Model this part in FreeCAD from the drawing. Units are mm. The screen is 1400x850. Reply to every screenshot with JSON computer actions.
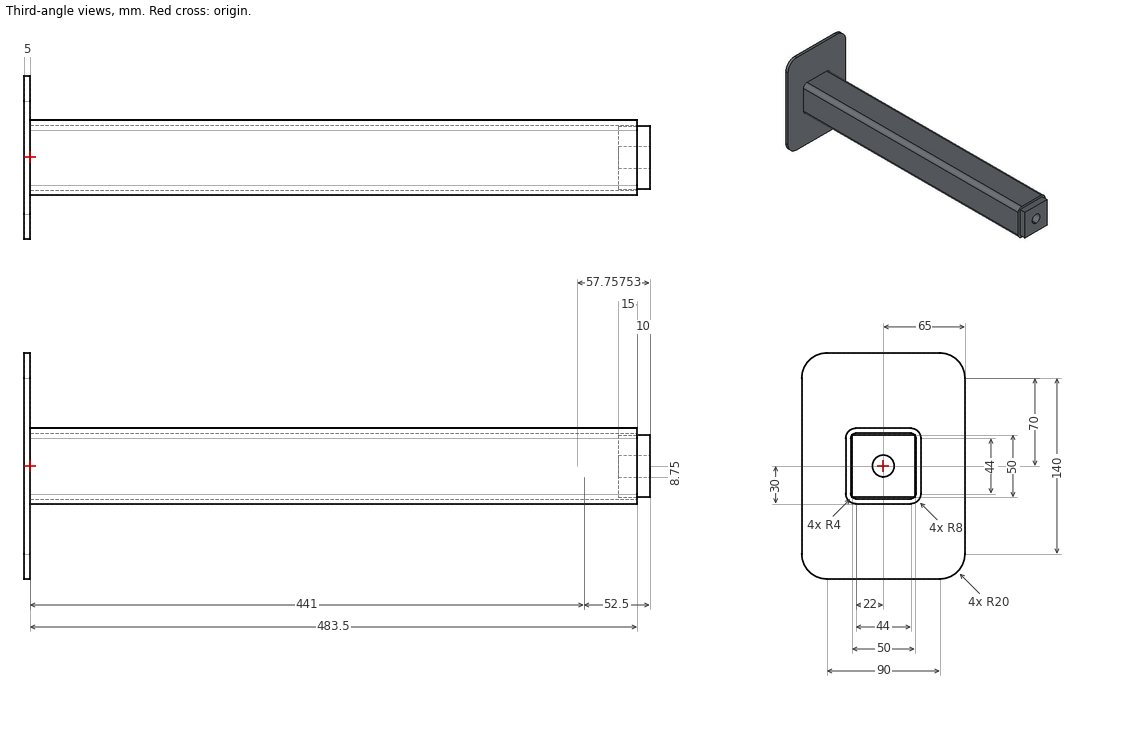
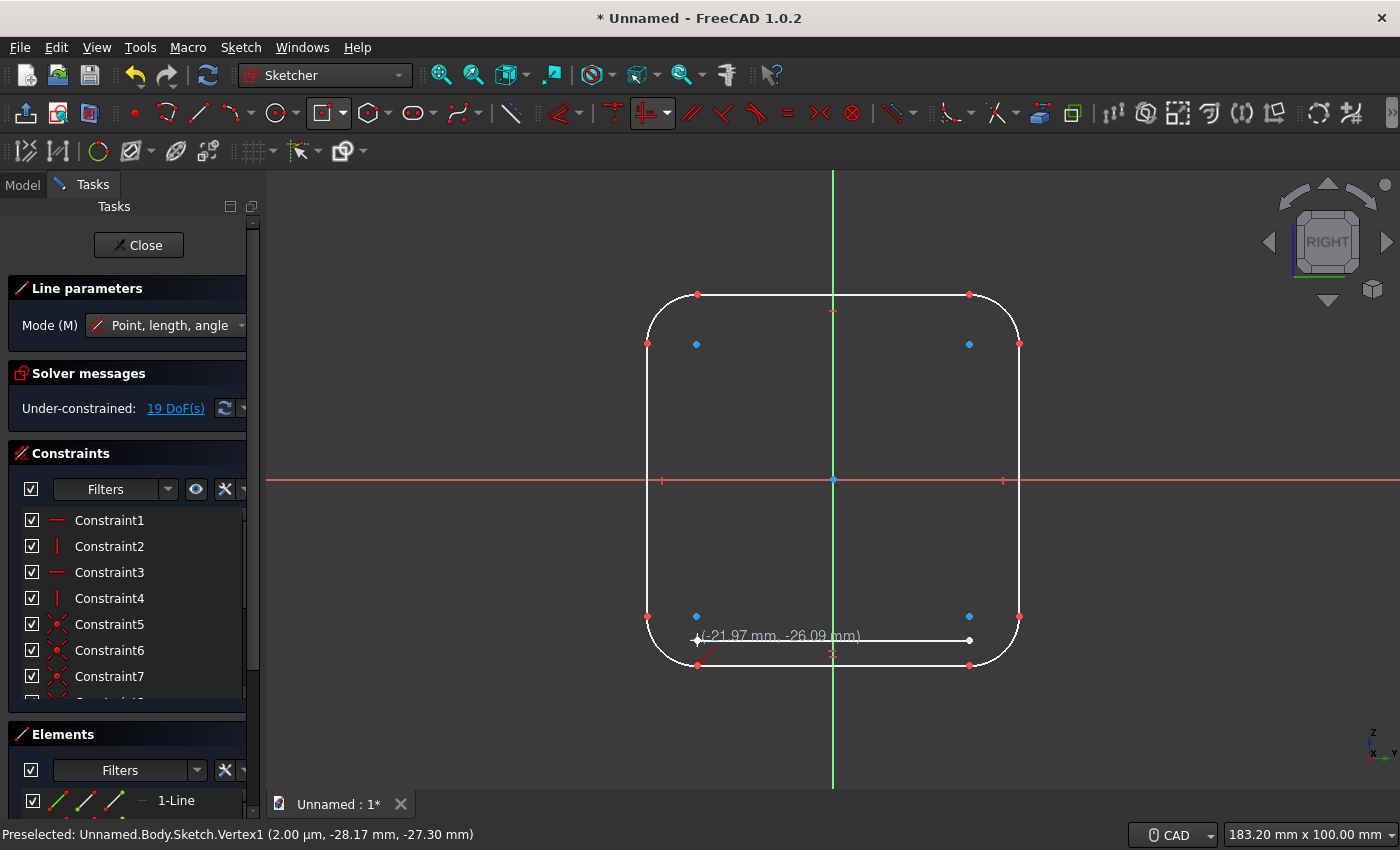
{"action": "left_click", "coordinate": [672, 616]}
{"action": "left_click", "coordinate": [672, 343]}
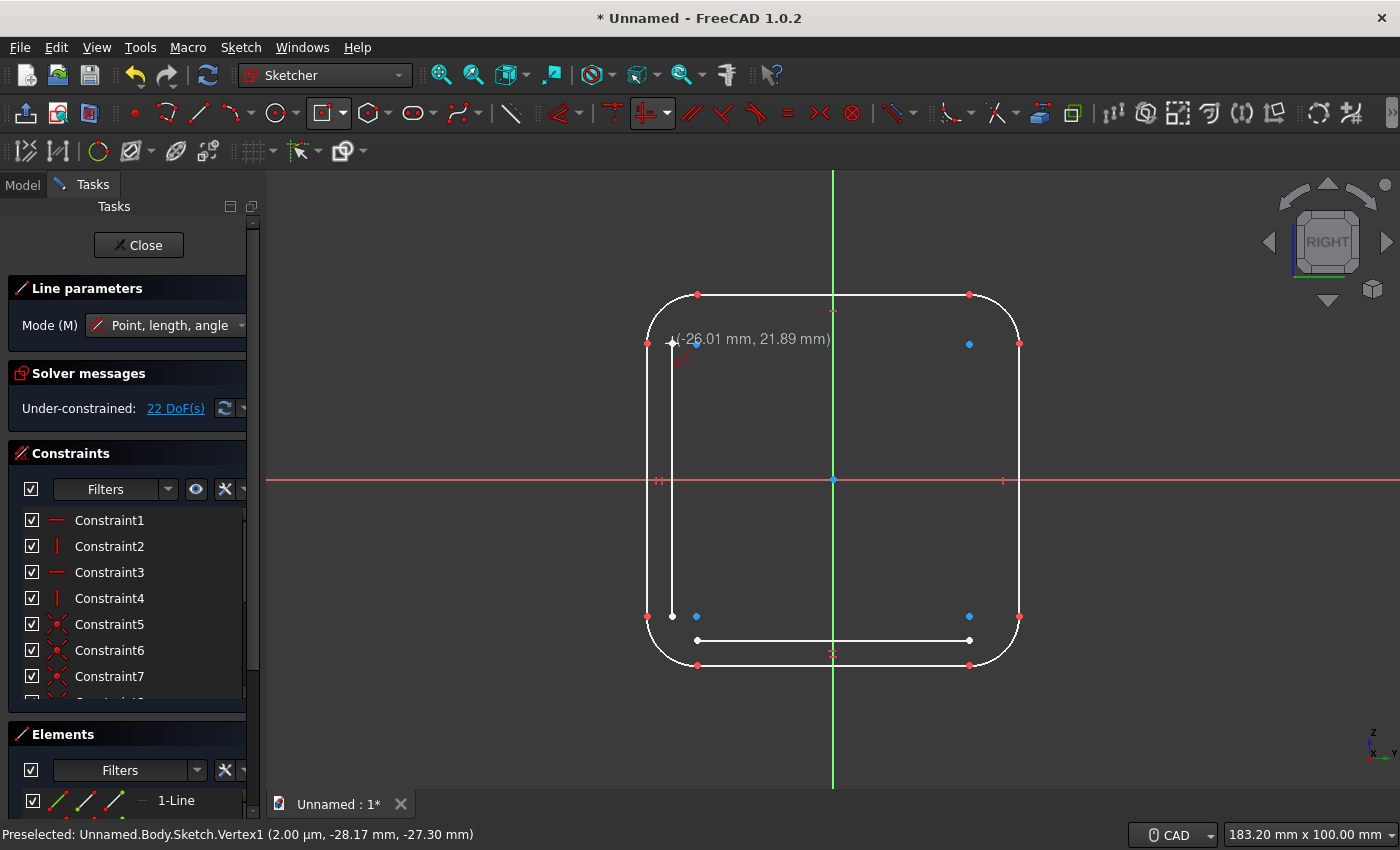
{"action": "left_click", "coordinate": [697, 319]}
{"action": "left_click", "coordinate": [969, 319]}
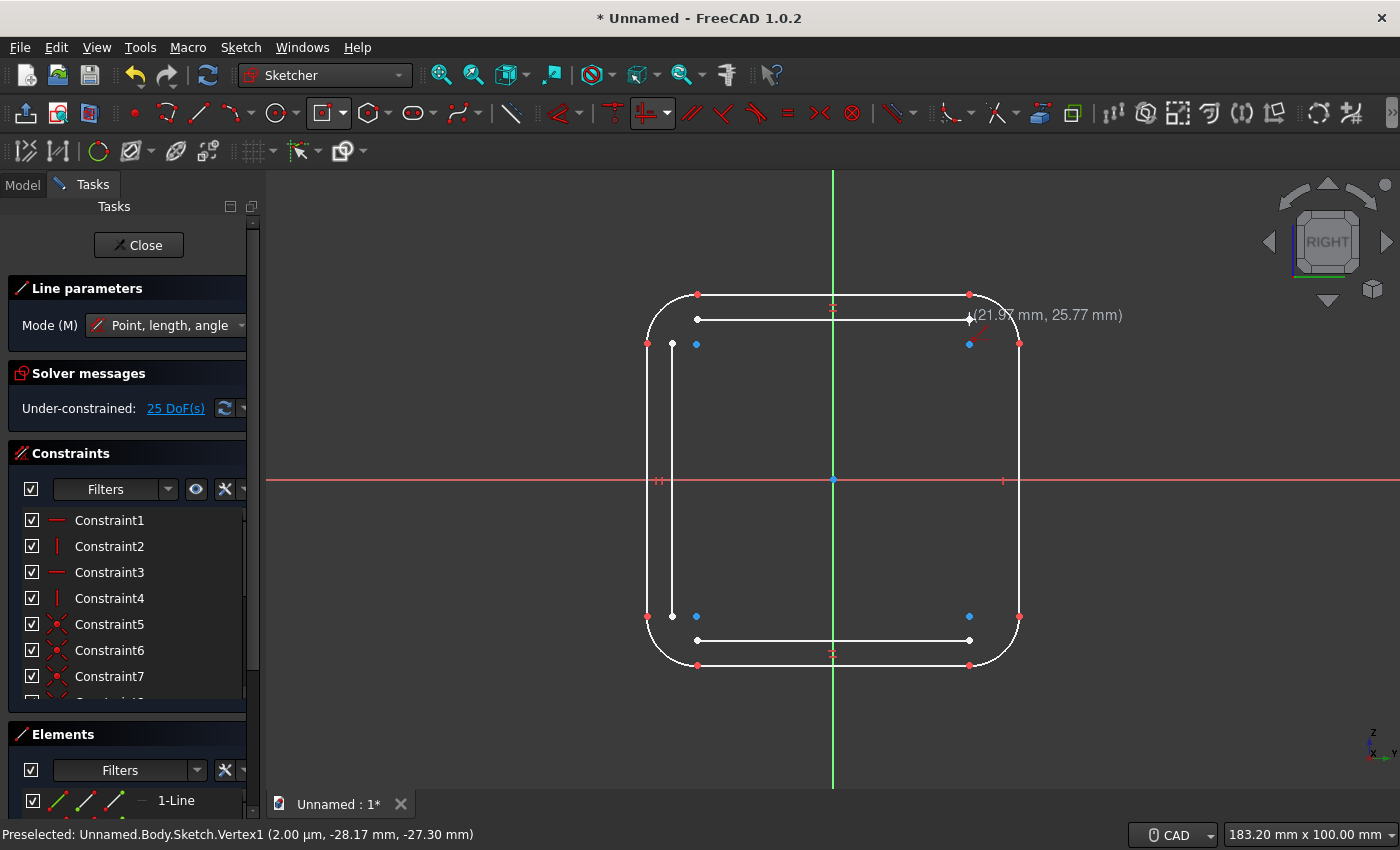
{"action": "left_click", "coordinate": [994, 343]}
{"action": "left_click", "coordinate": [994, 616]}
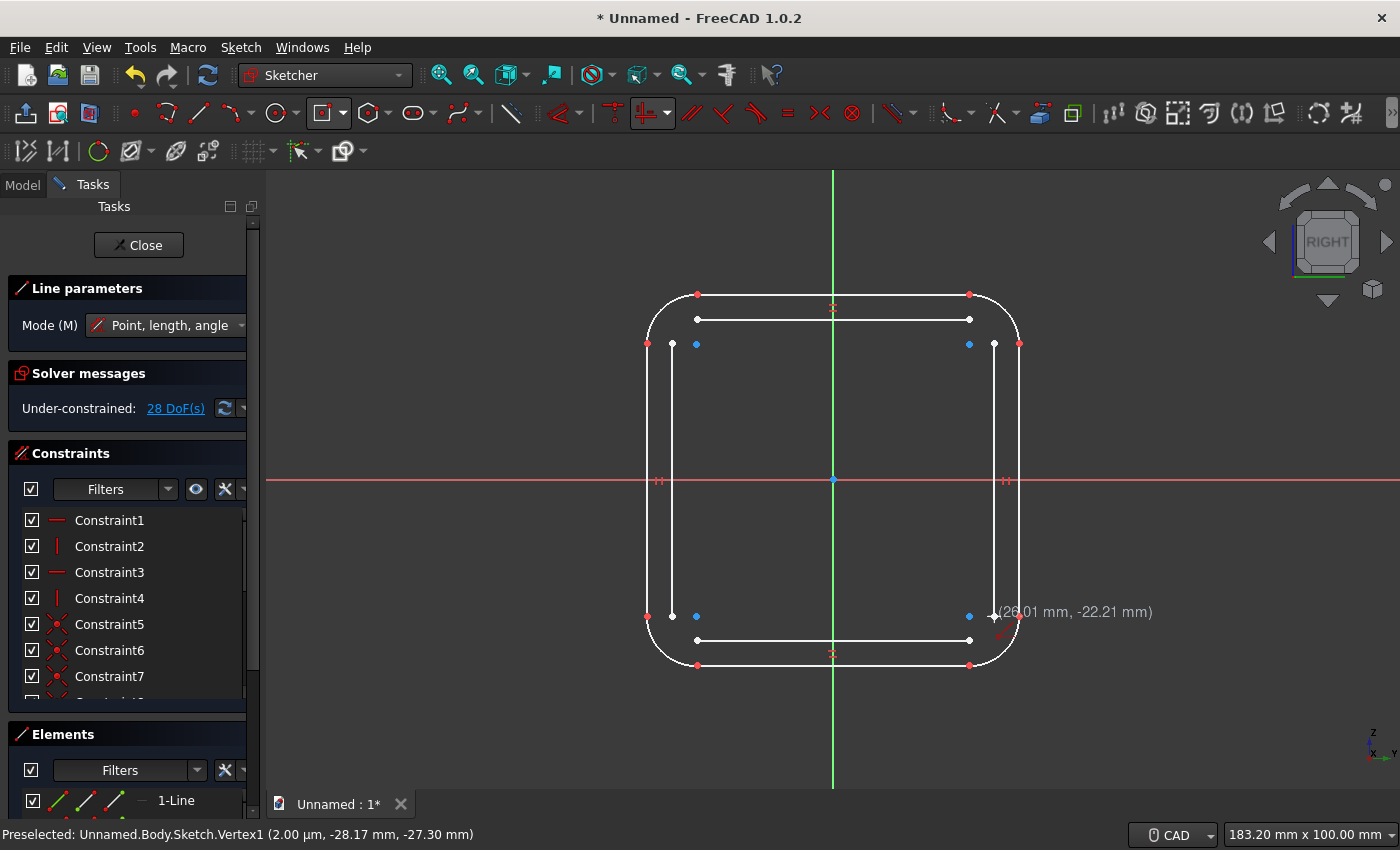
{"action": "left_click", "coordinate": [232, 114]}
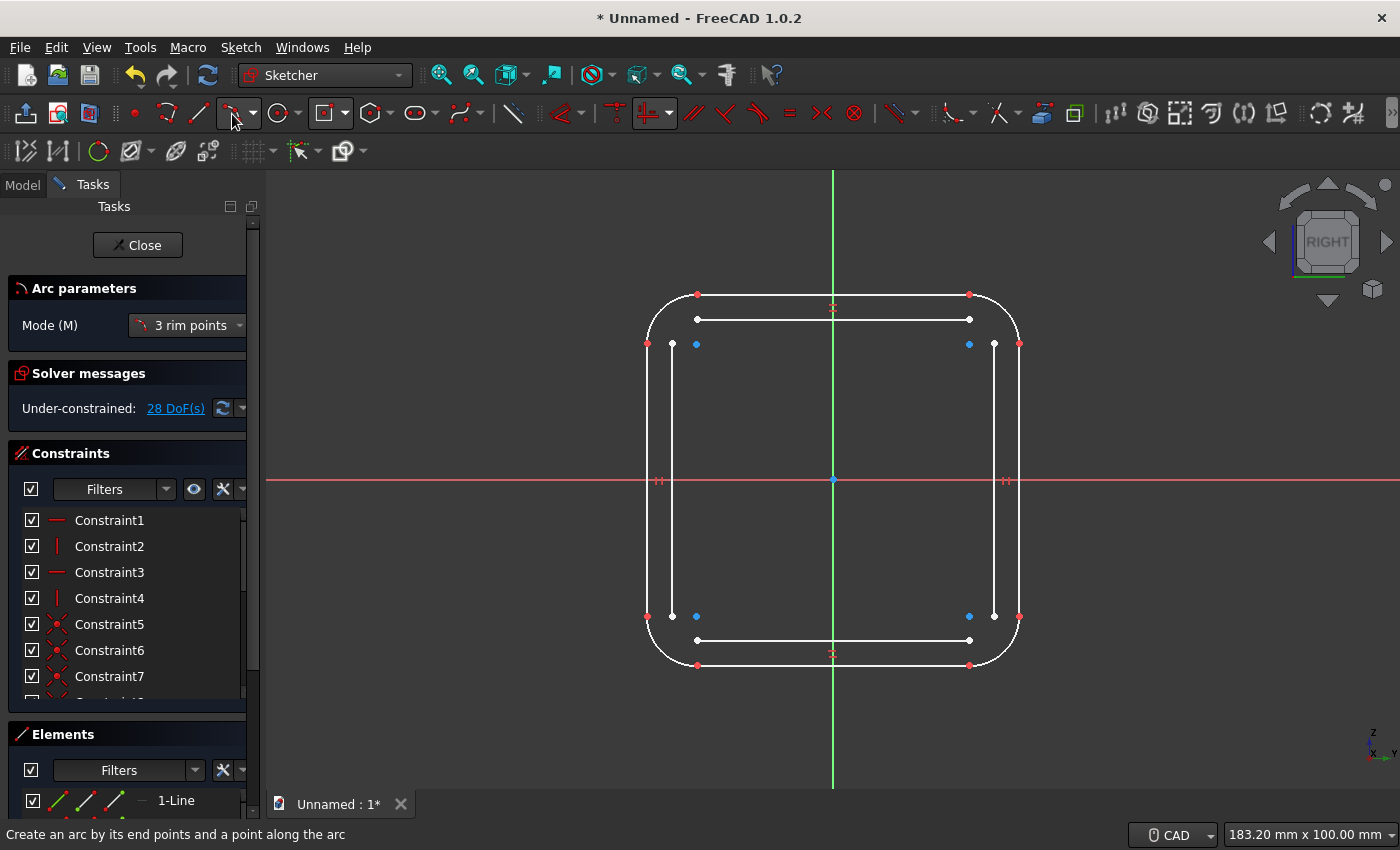
{"action": "left_click", "coordinate": [697, 641]}
{"action": "left_click", "coordinate": [672, 617]}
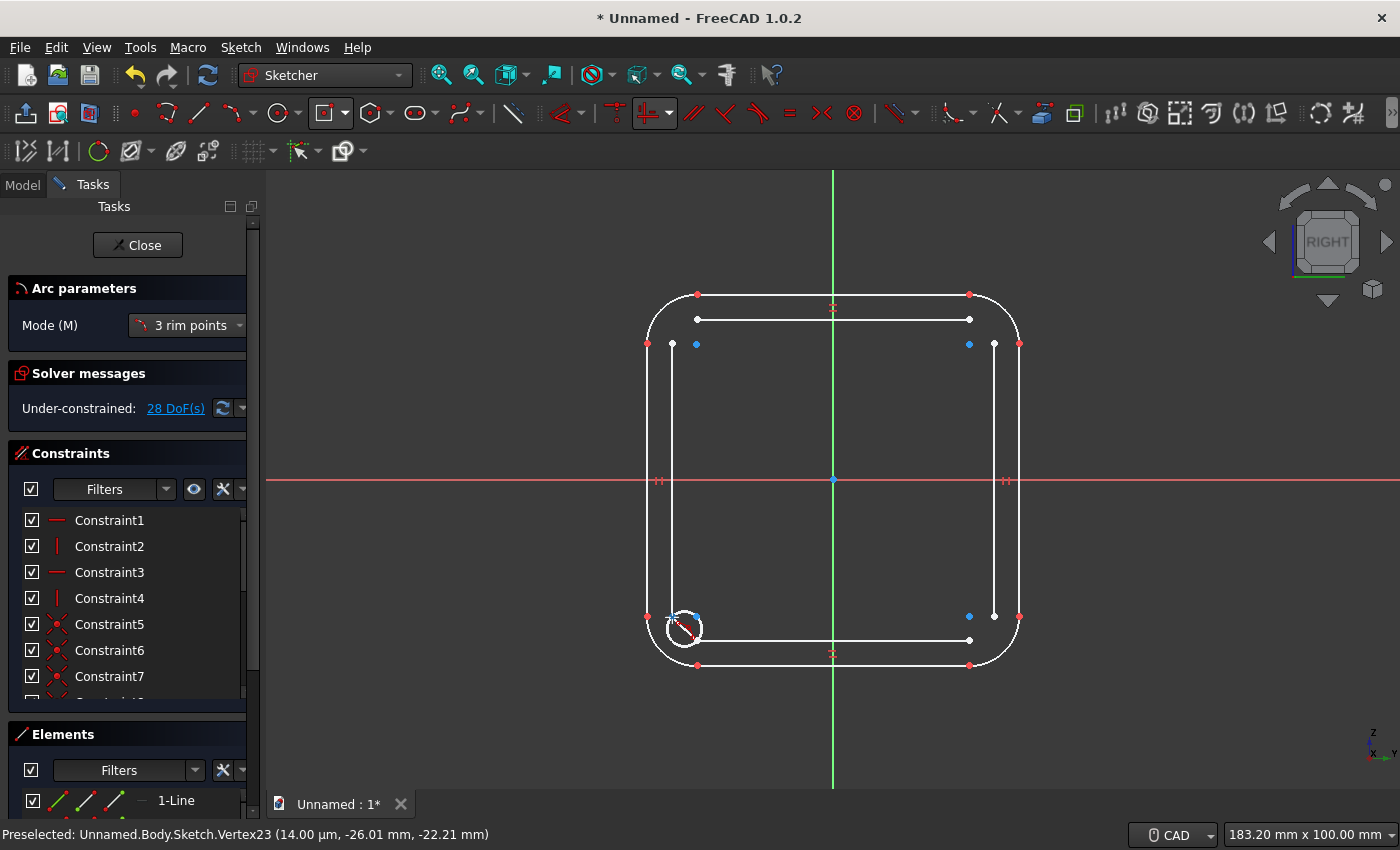
{"action": "scroll", "coordinate": [679, 633], "scroll_direction": "up", "scroll_amount": 4}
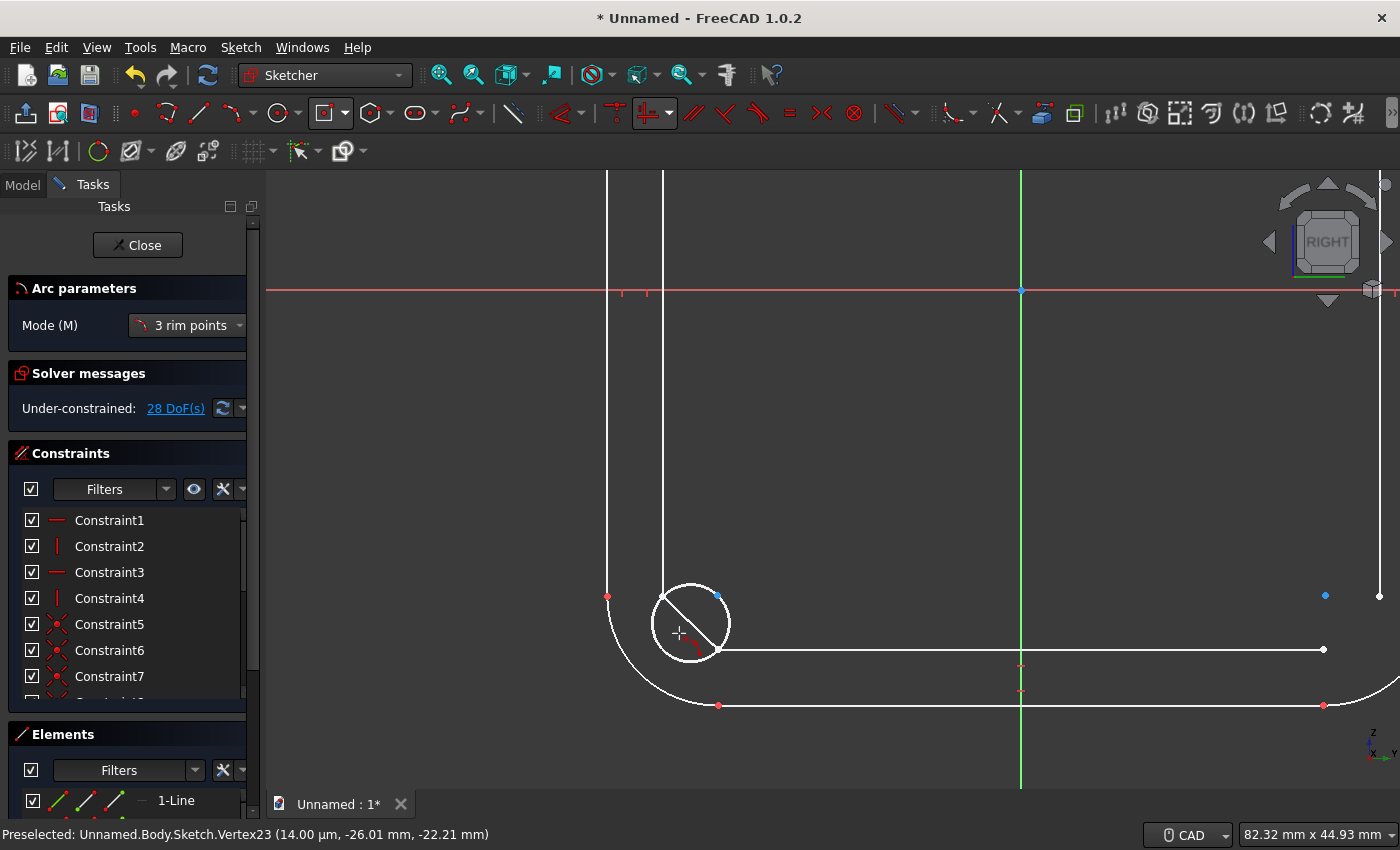
{"action": "left_click", "coordinate": [679, 633]}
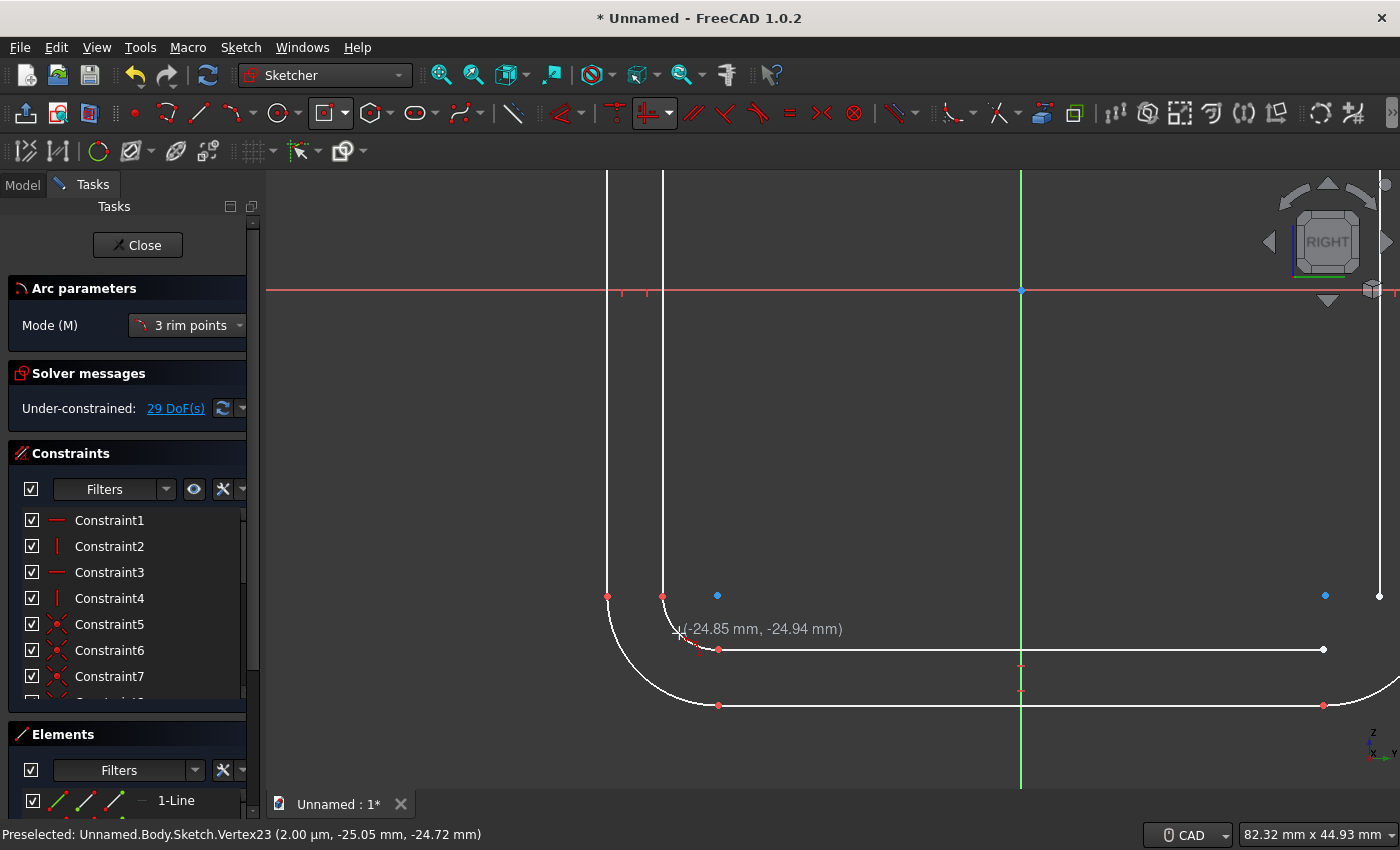
{"action": "scroll", "coordinate": [555, 634], "scroll_direction": "down", "scroll_amount": 4}